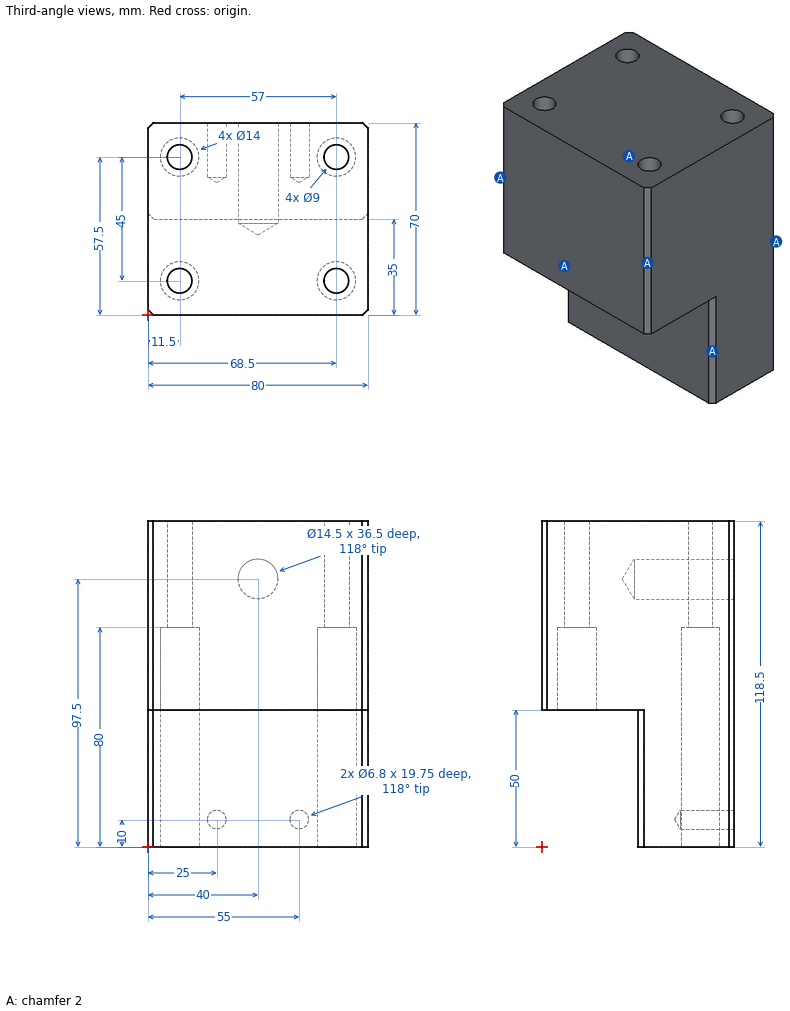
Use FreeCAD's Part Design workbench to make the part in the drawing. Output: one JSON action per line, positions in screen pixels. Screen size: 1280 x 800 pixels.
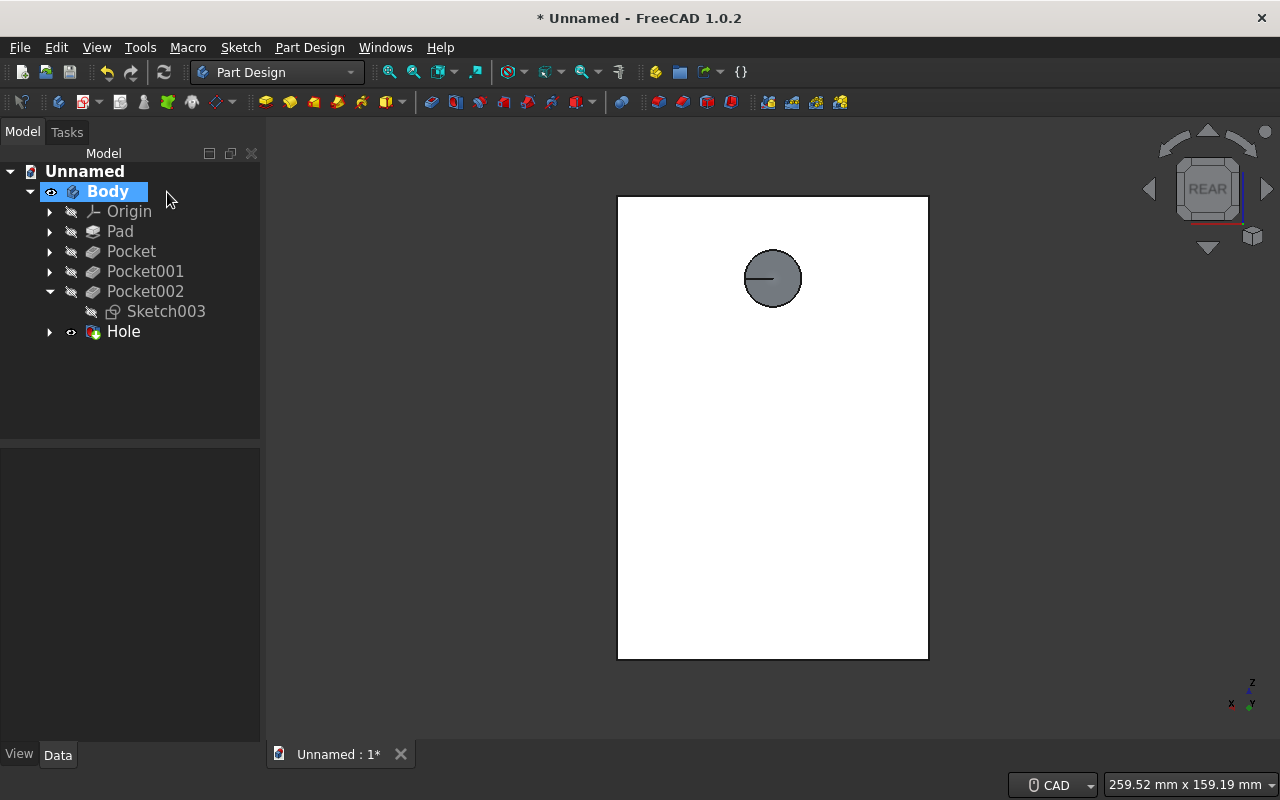
{"action": "left_click", "coordinate": [773, 493]}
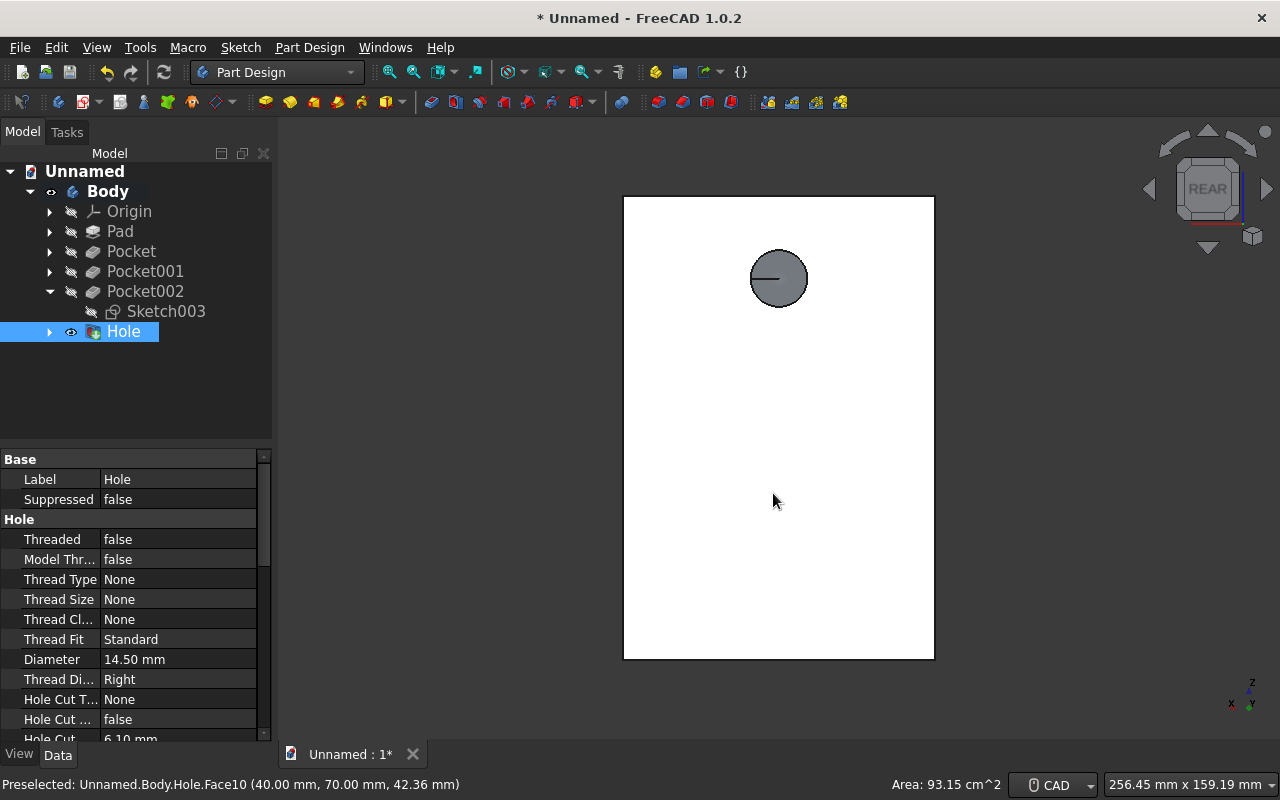
{"action": "left_click", "coordinate": [84, 102]}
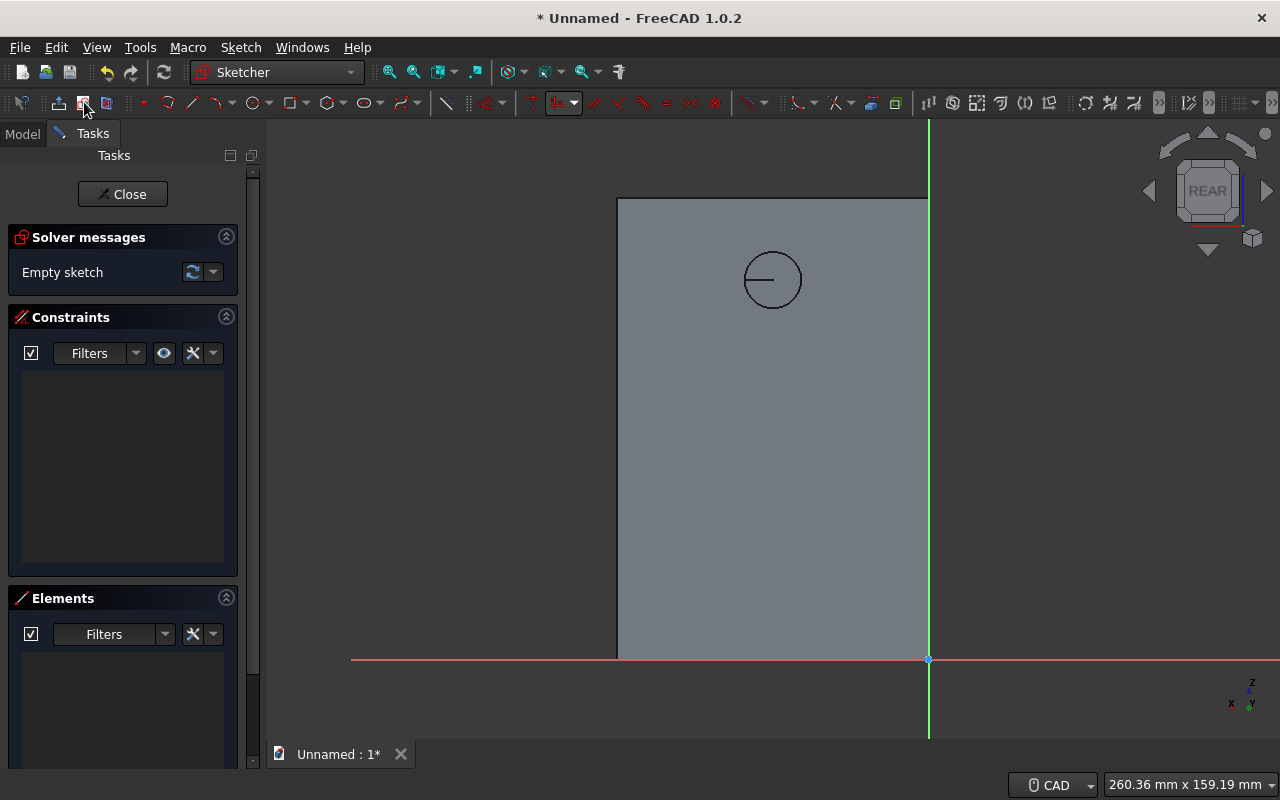
{"action": "scroll", "coordinate": [879, 711], "scroll_direction": "up", "scroll_amount": 5}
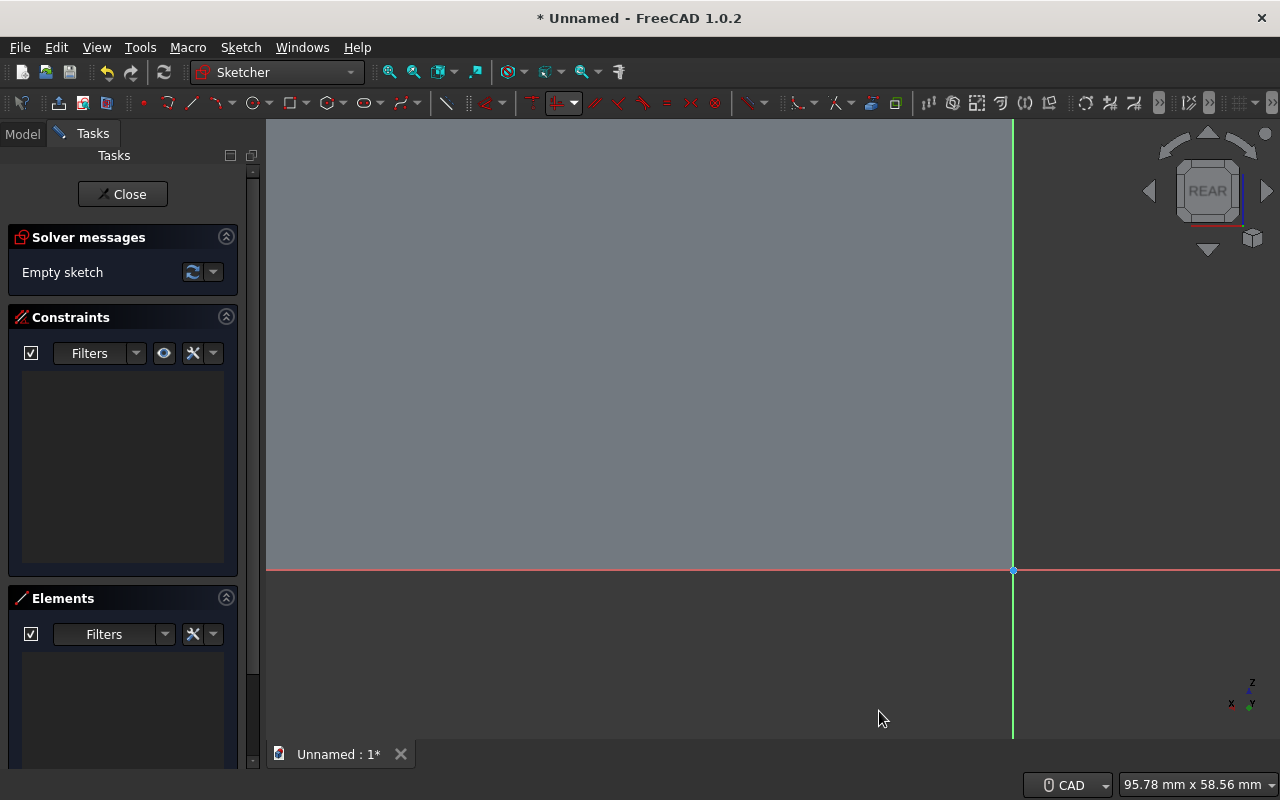
{"action": "key", "text": "g c"}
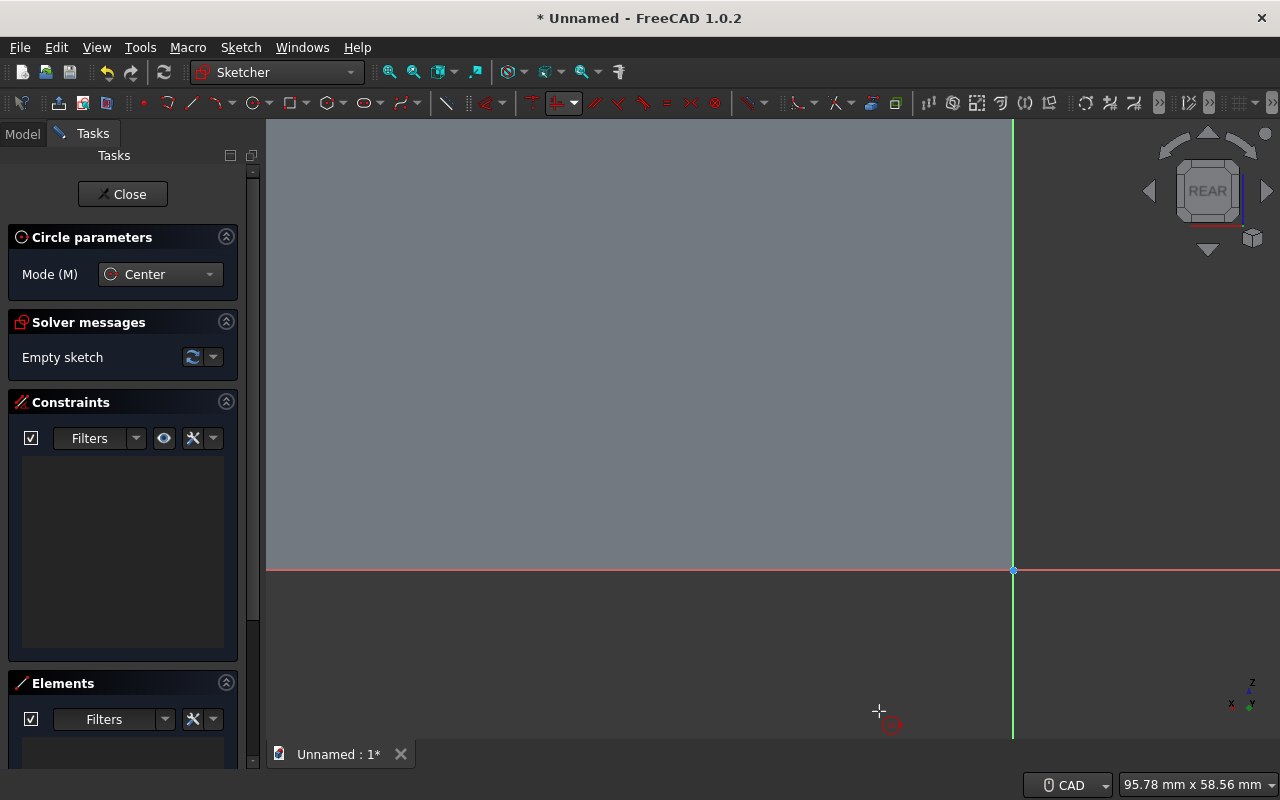
{"action": "left_click", "coordinate": [431, 464]}
{"action": "left_click", "coordinate": [456, 439]}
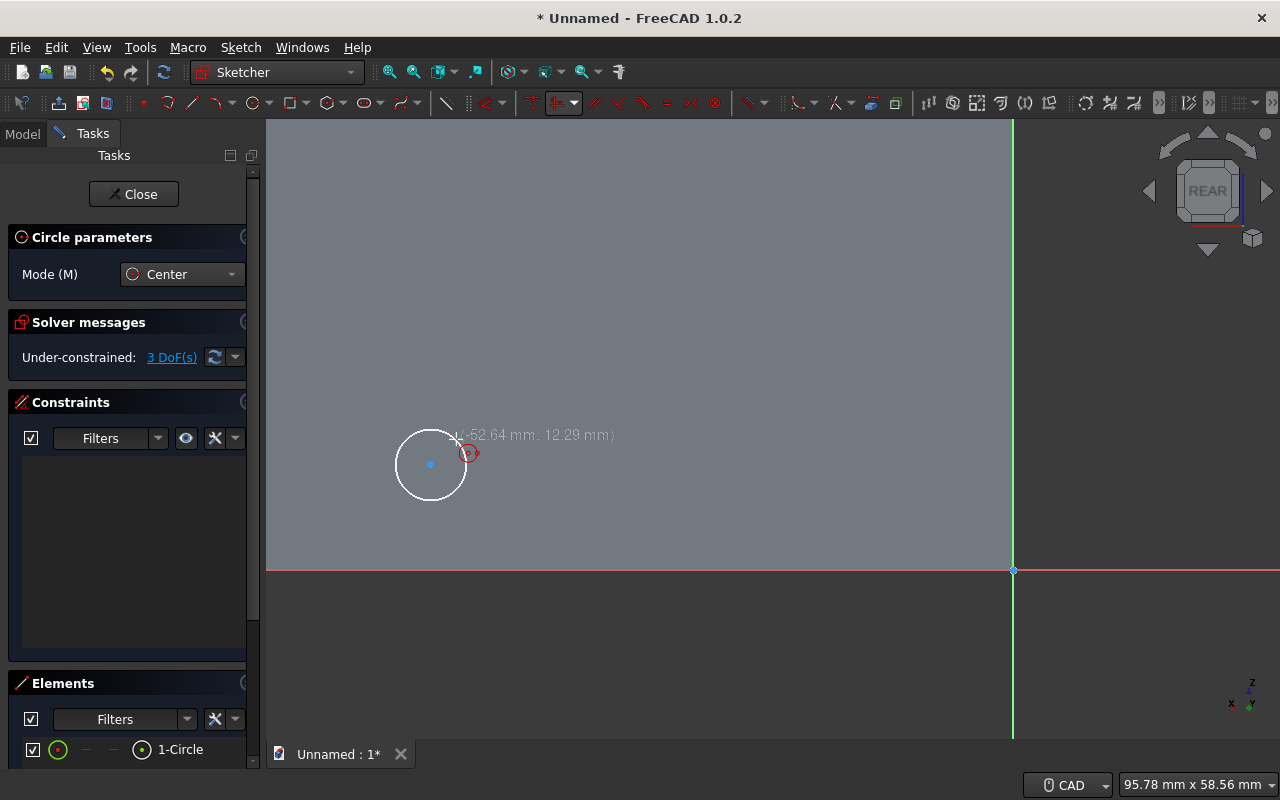
{"action": "left_click", "coordinate": [749, 464]}
{"action": "left_click", "coordinate": [774, 439]}
{"action": "key", "text": "Escape"}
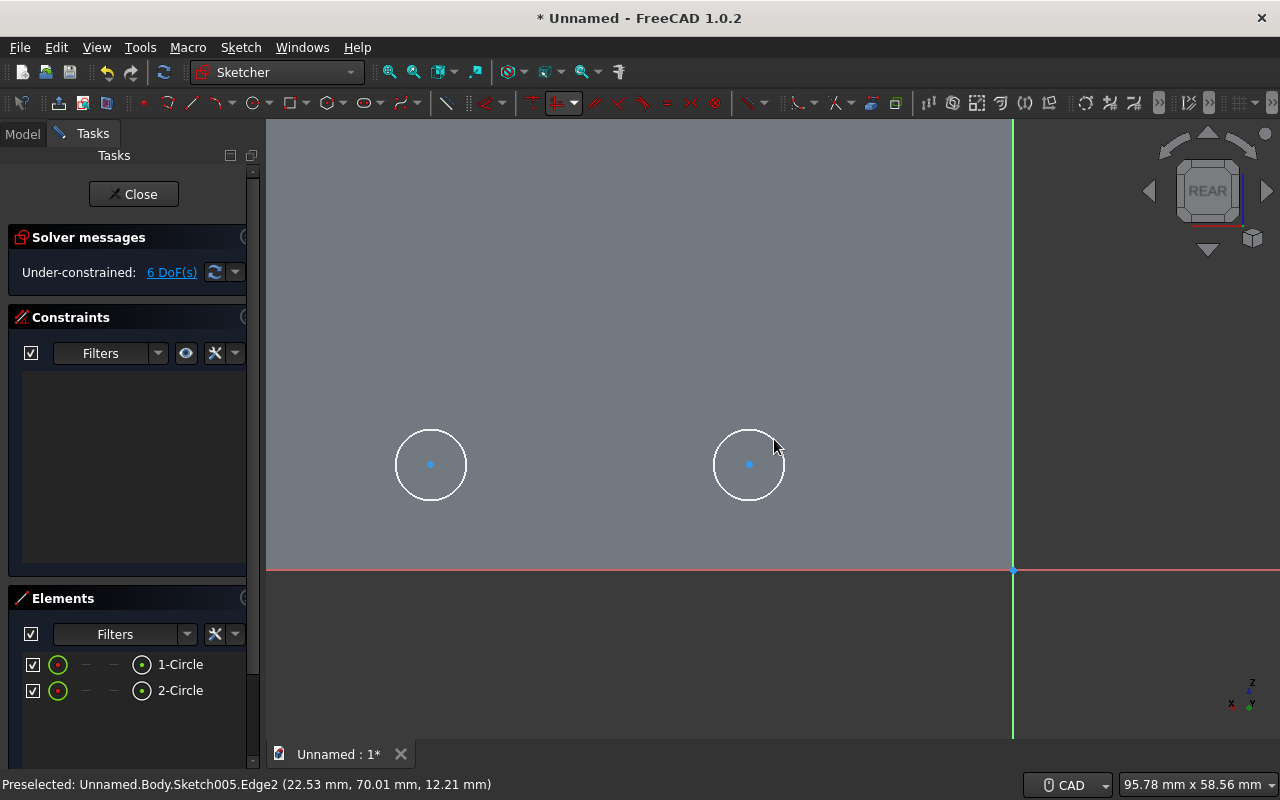
{"action": "left_click", "coordinate": [456, 440]}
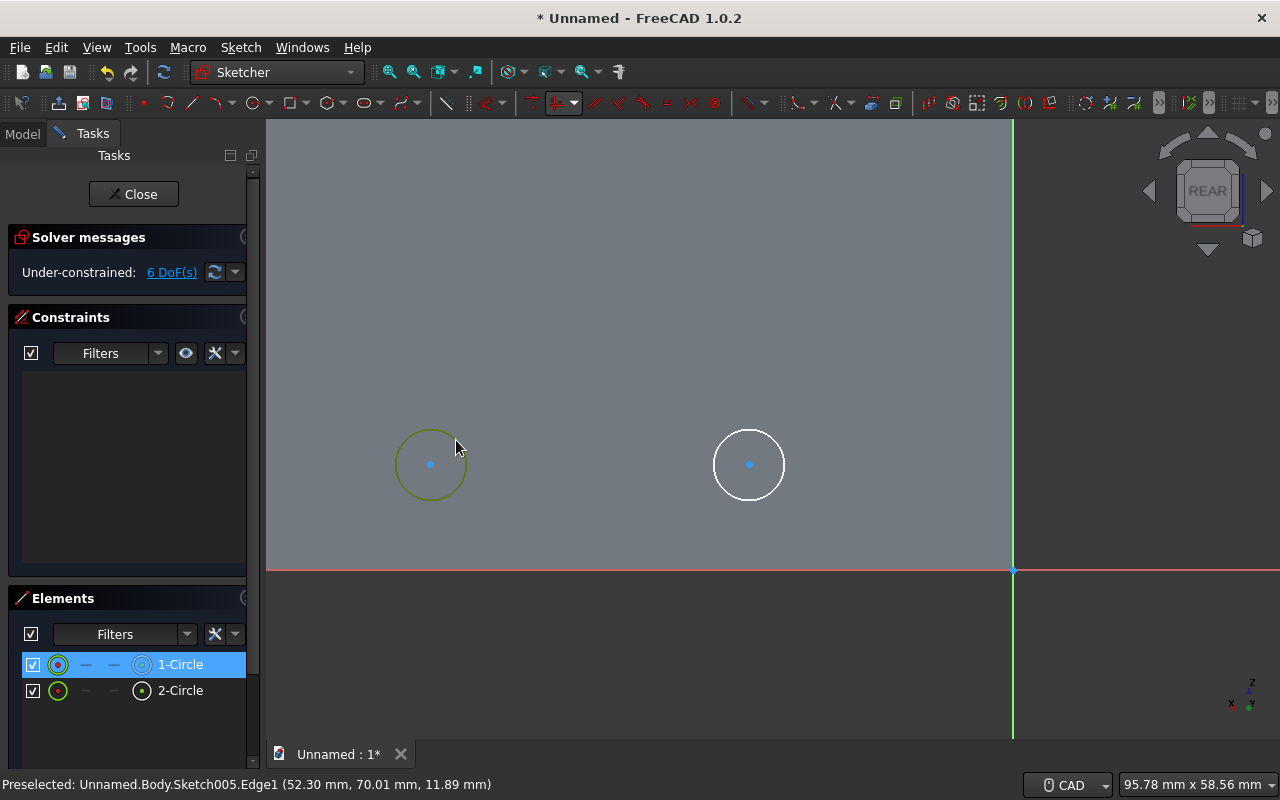
{"action": "left_click", "coordinate": [774, 440]}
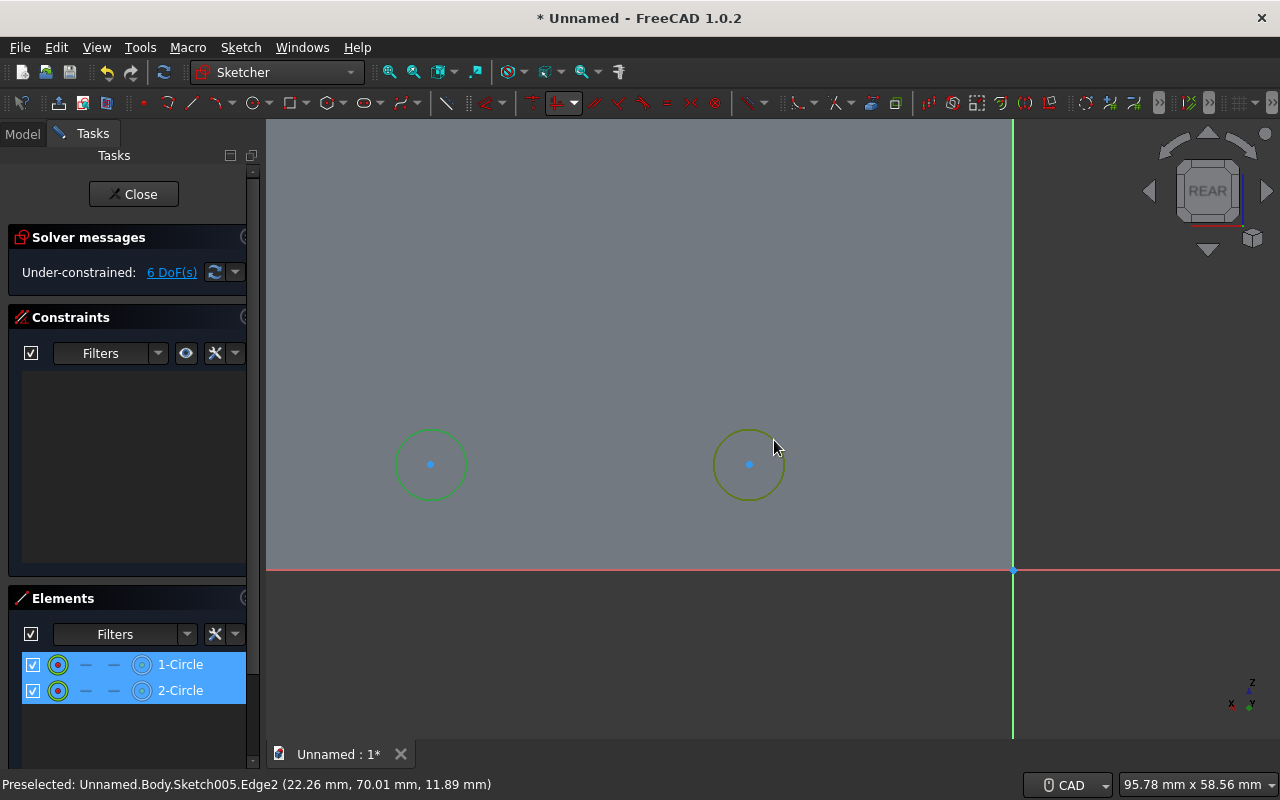
{"action": "key", "text": "e"}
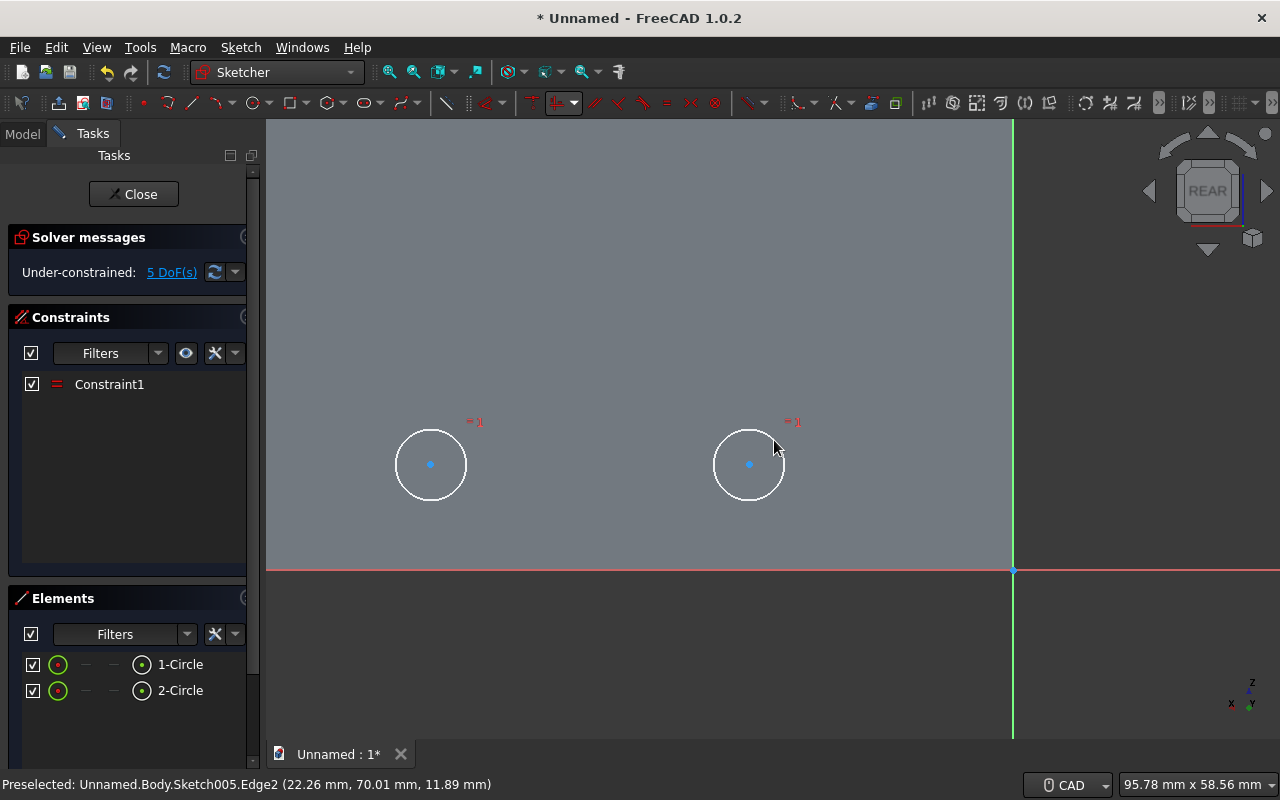
{"action": "left_click", "coordinate": [431, 465]}